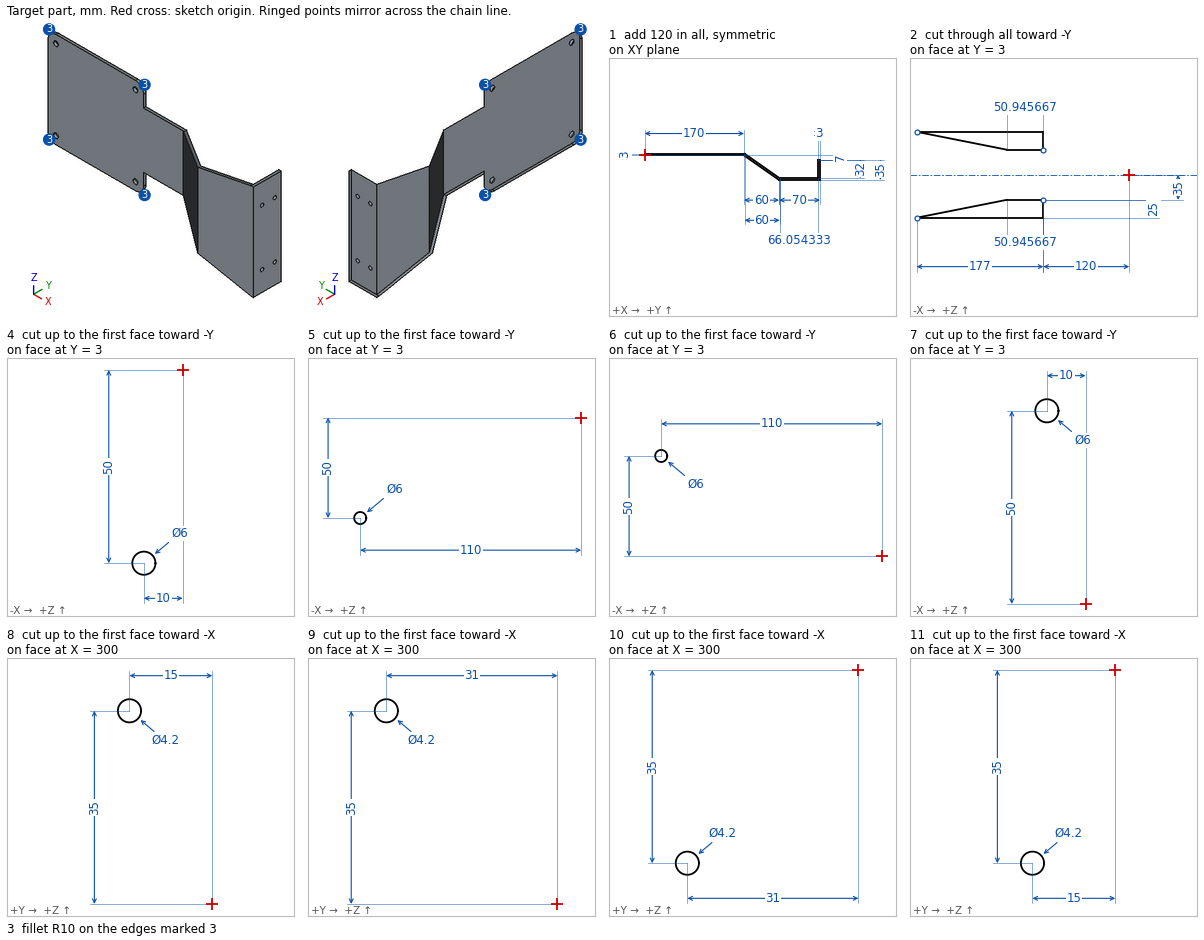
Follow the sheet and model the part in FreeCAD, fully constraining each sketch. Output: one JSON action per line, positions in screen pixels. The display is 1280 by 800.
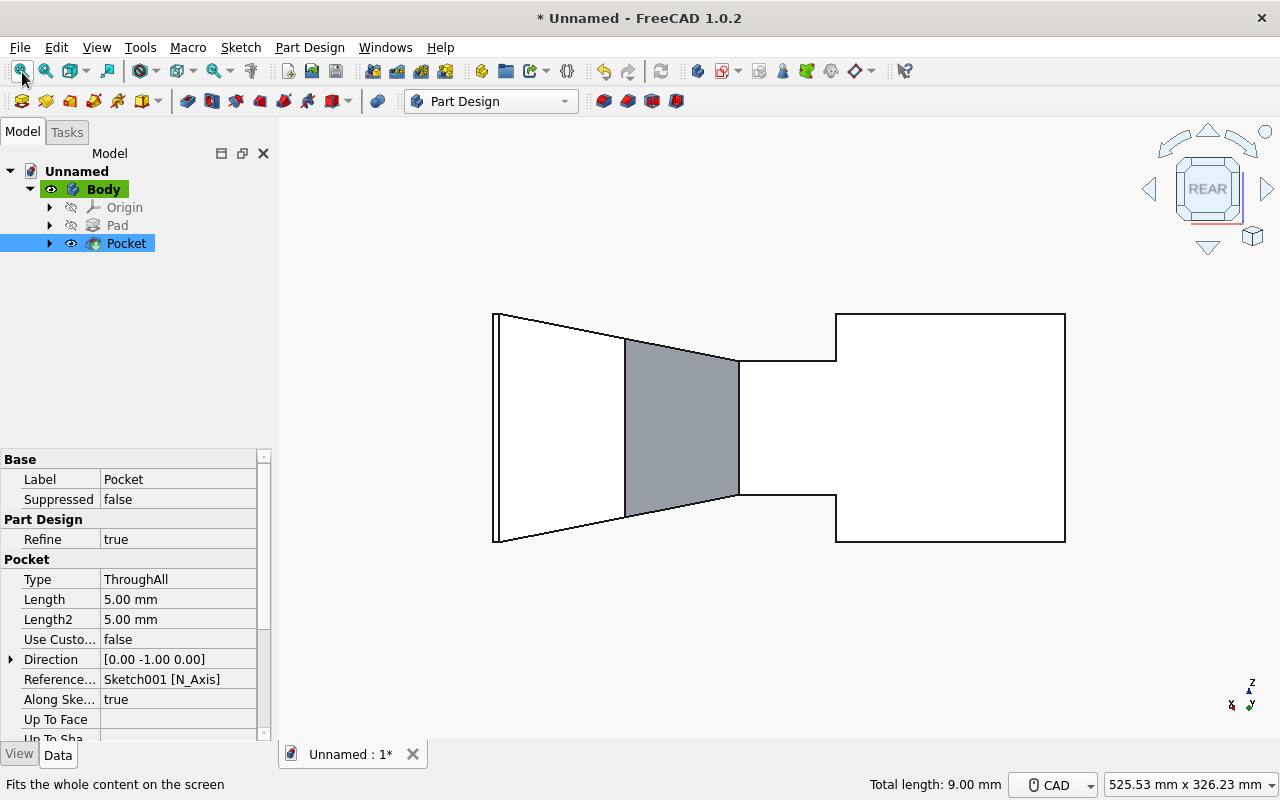
{"action": "scroll", "coordinate": [836, 313], "scroll_direction": "up", "scroll_amount": 10}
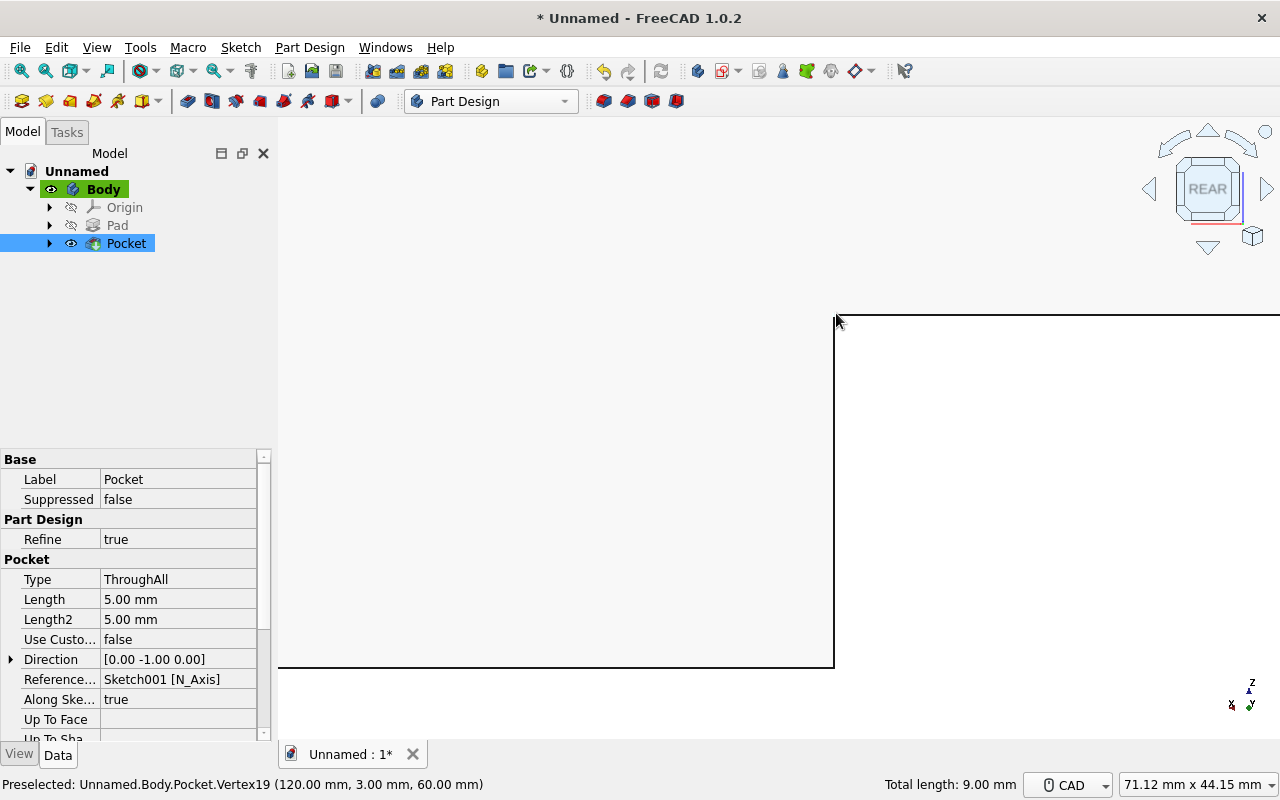
{"action": "left_click", "coordinate": [22, 72]}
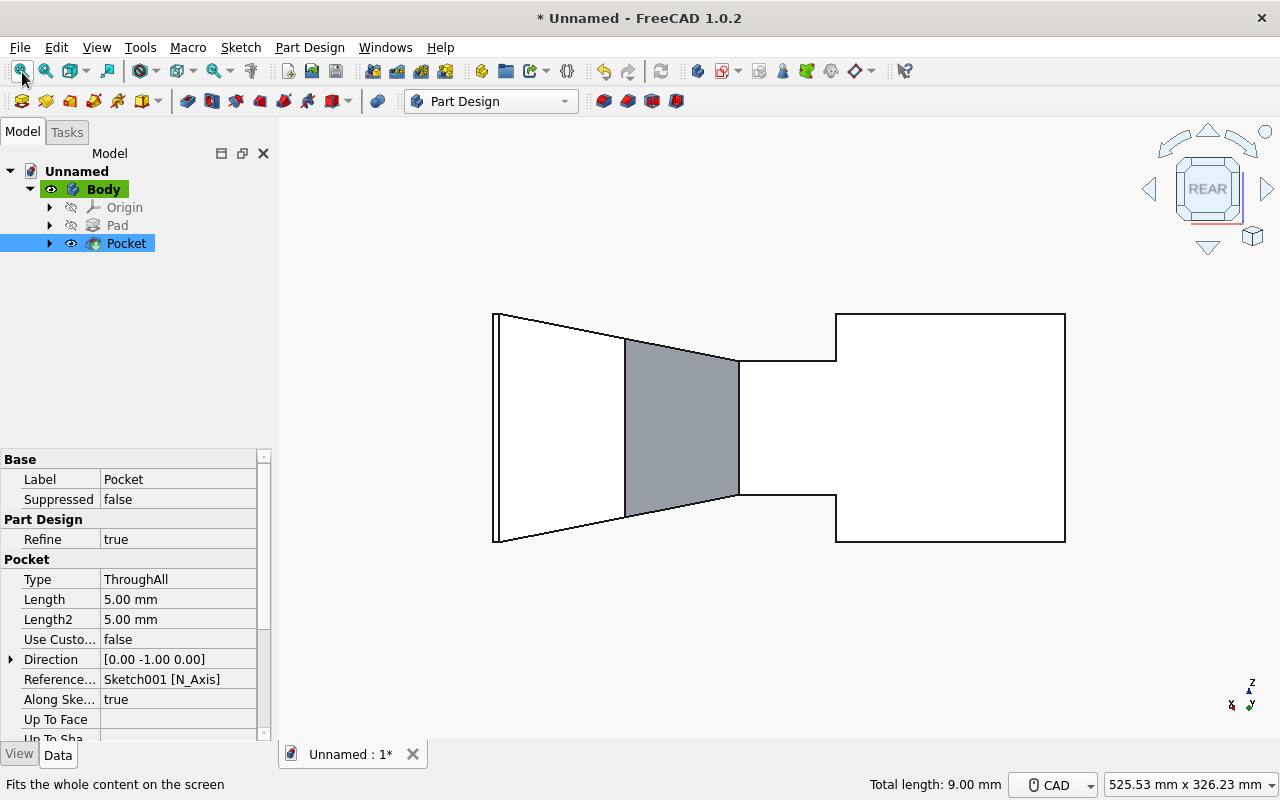
{"action": "key", "text": "6"}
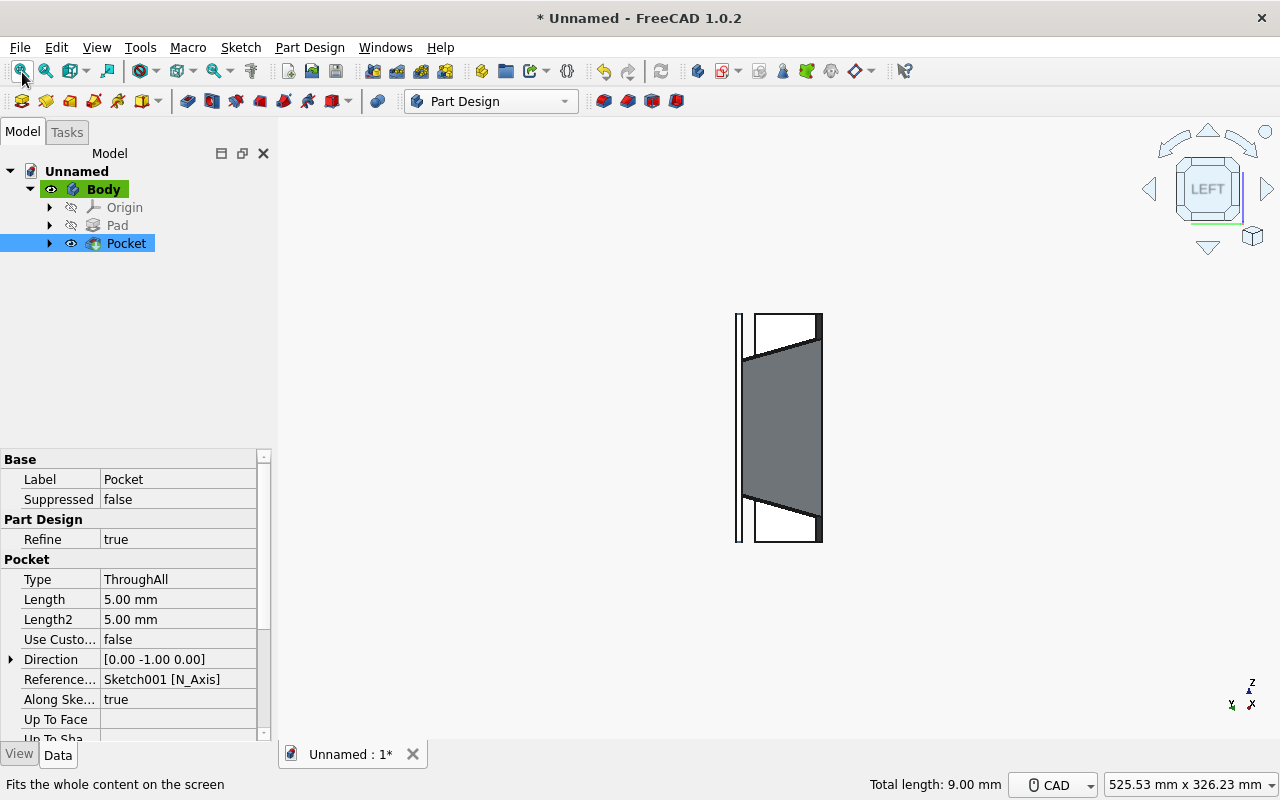
{"action": "left_click", "coordinate": [22, 72]}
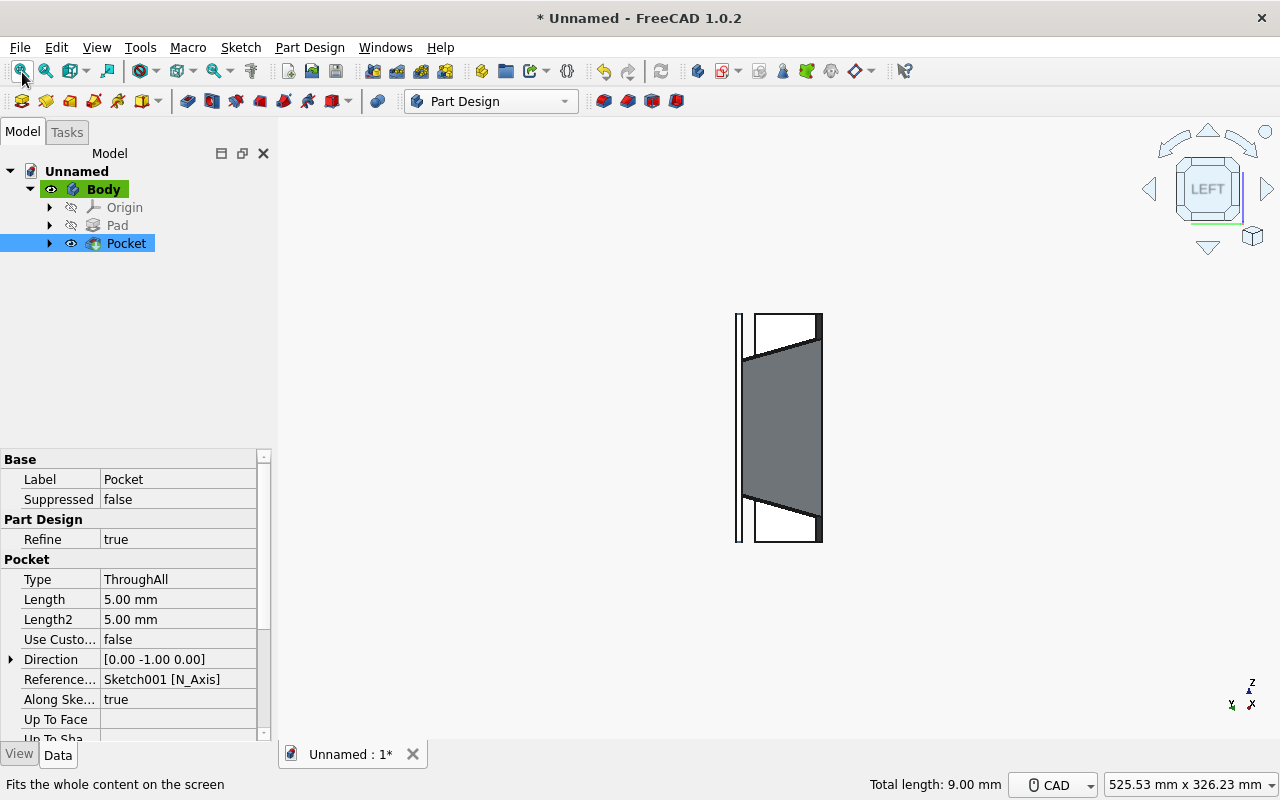
{"action": "scroll", "coordinate": [739, 313], "scroll_direction": "up", "scroll_amount": 10}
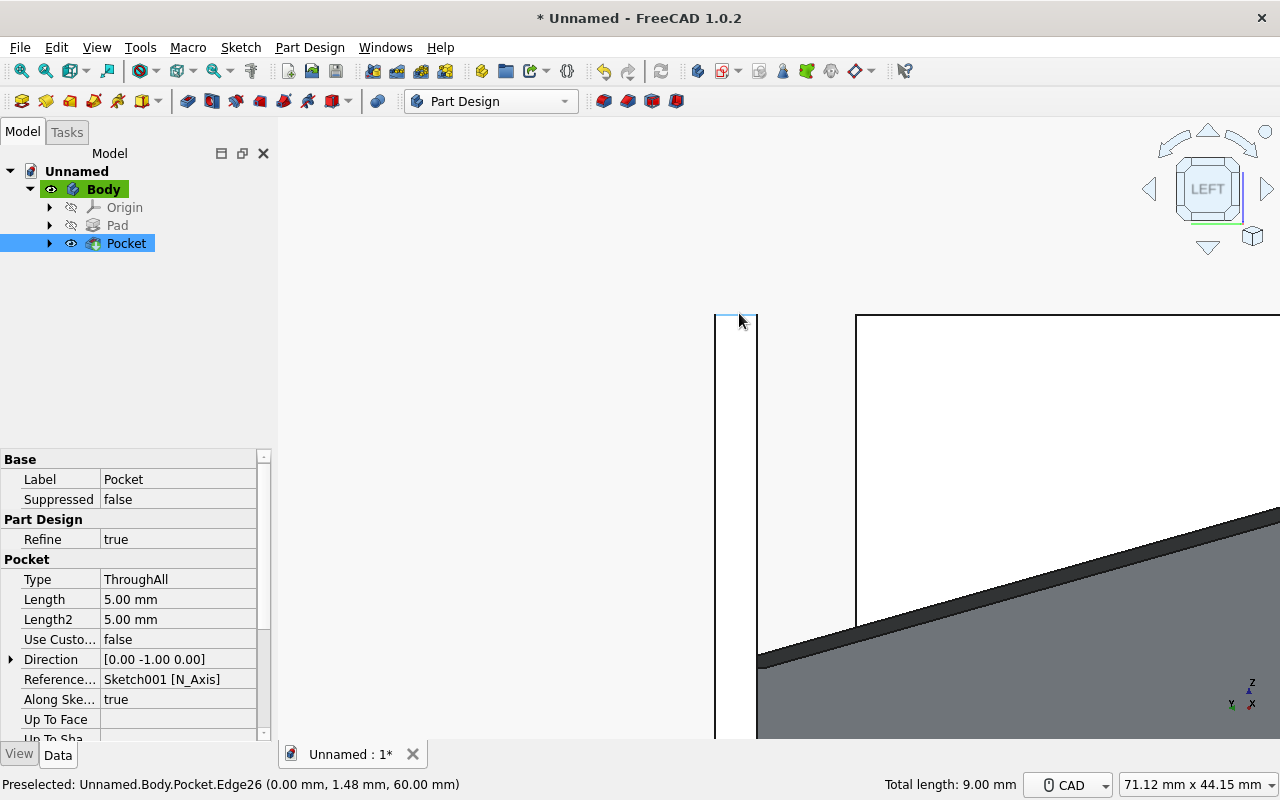
{"action": "left_click", "coordinate": [22, 72]}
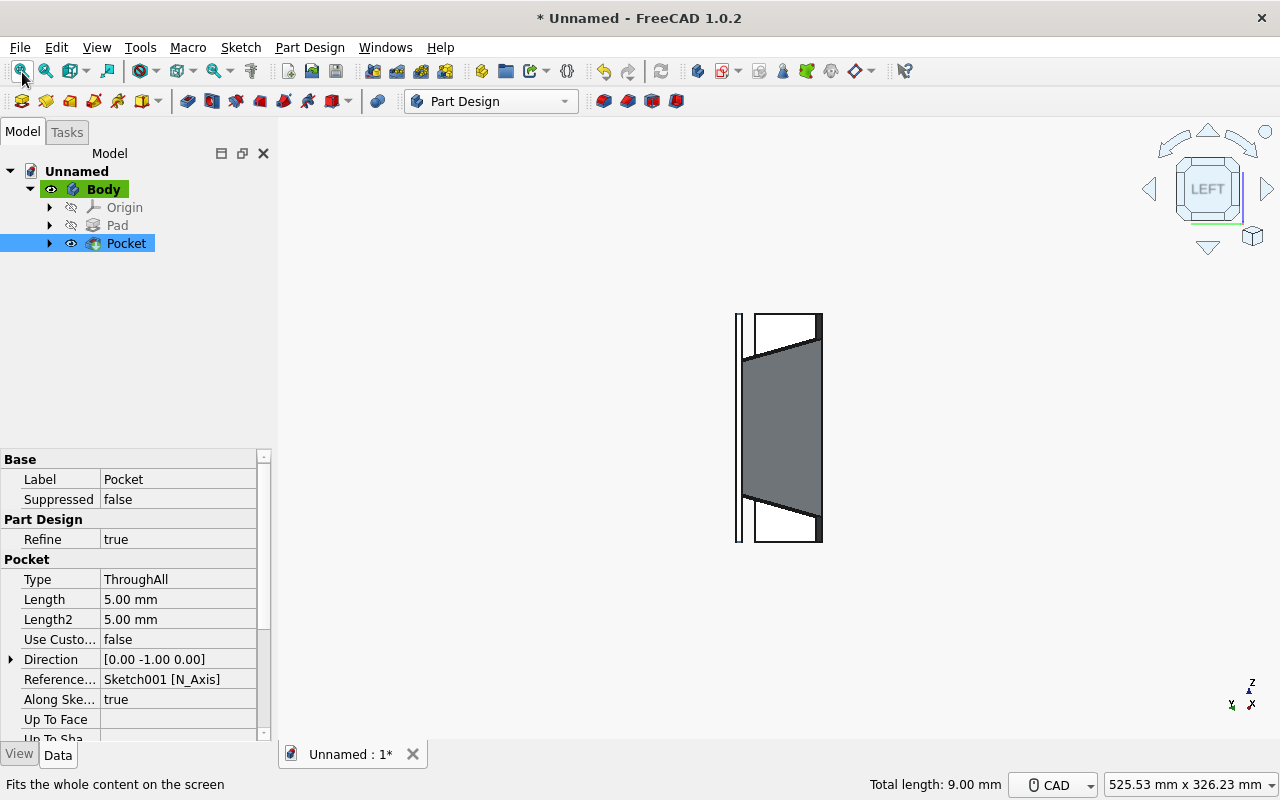
{"action": "key", "text": "v 3"}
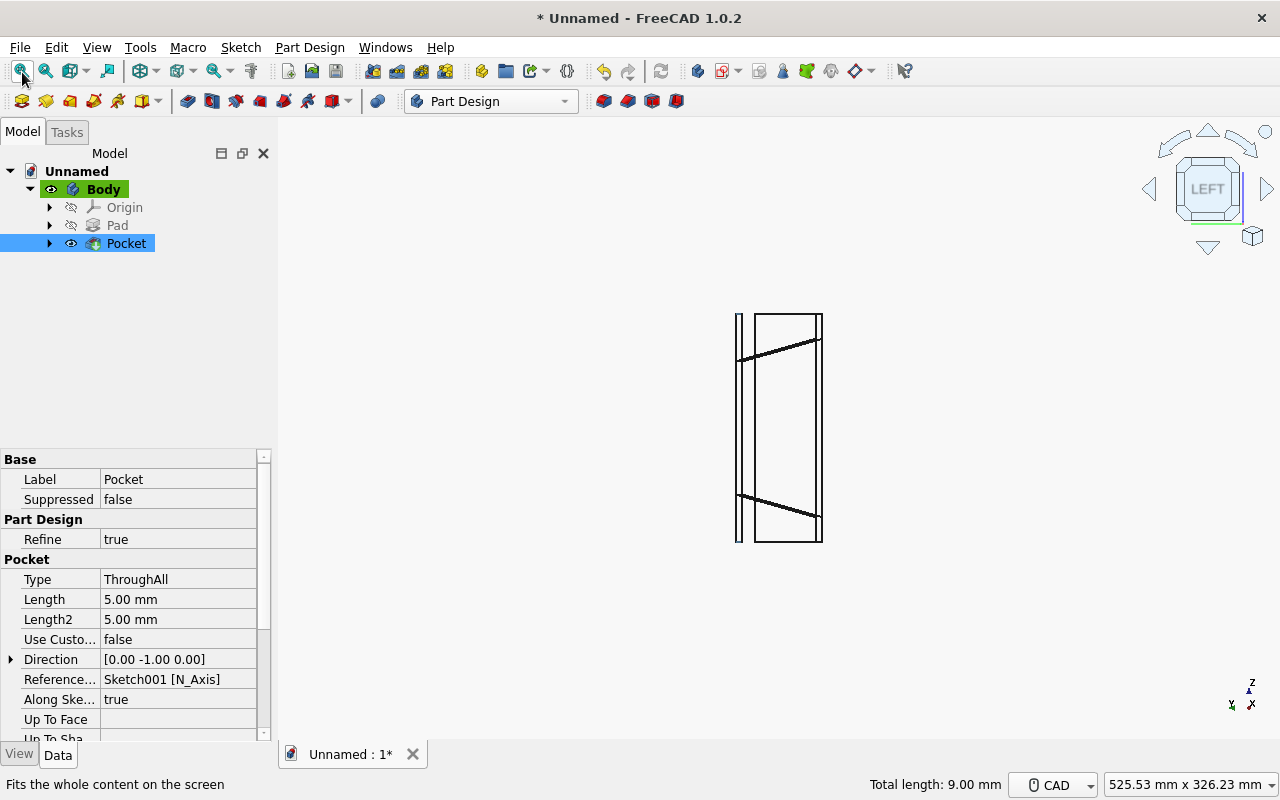
{"action": "key", "text": "0"}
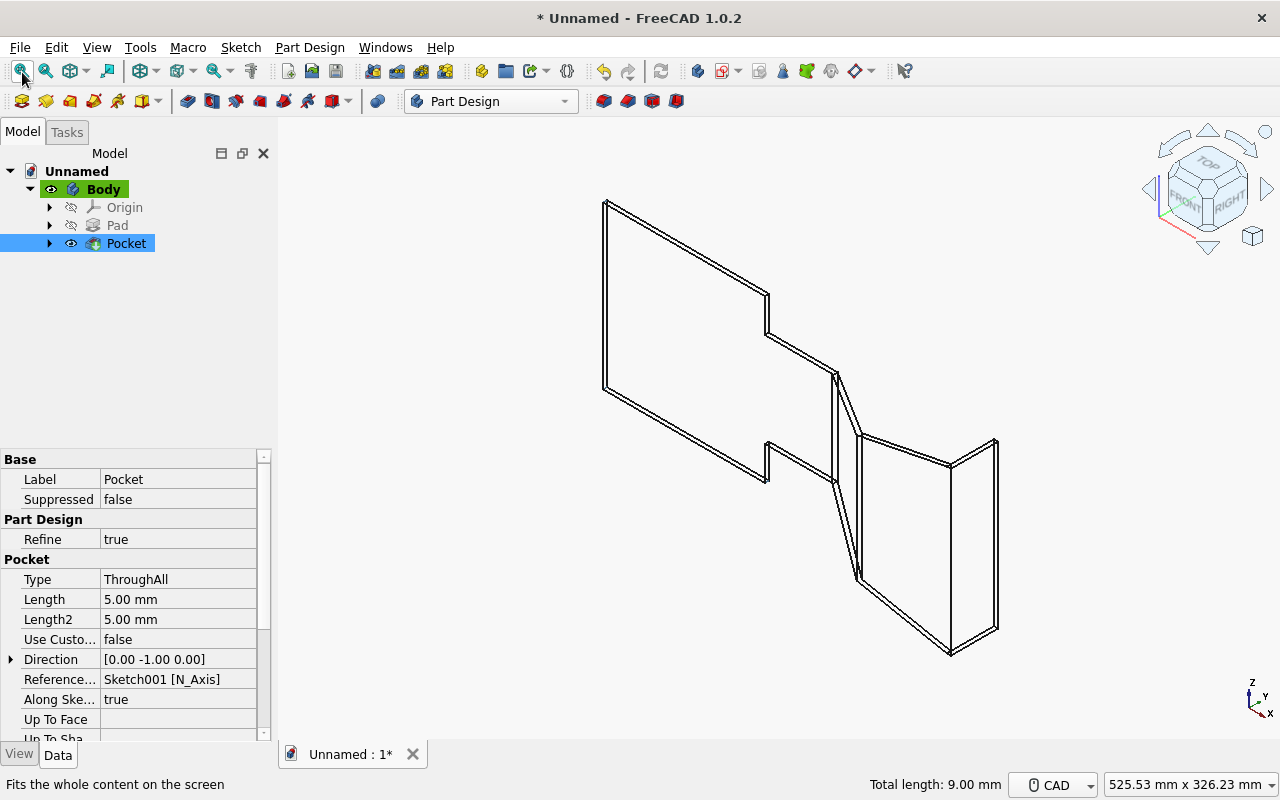
{"action": "scroll", "coordinate": [767, 294], "scroll_direction": "up", "scroll_amount": 10}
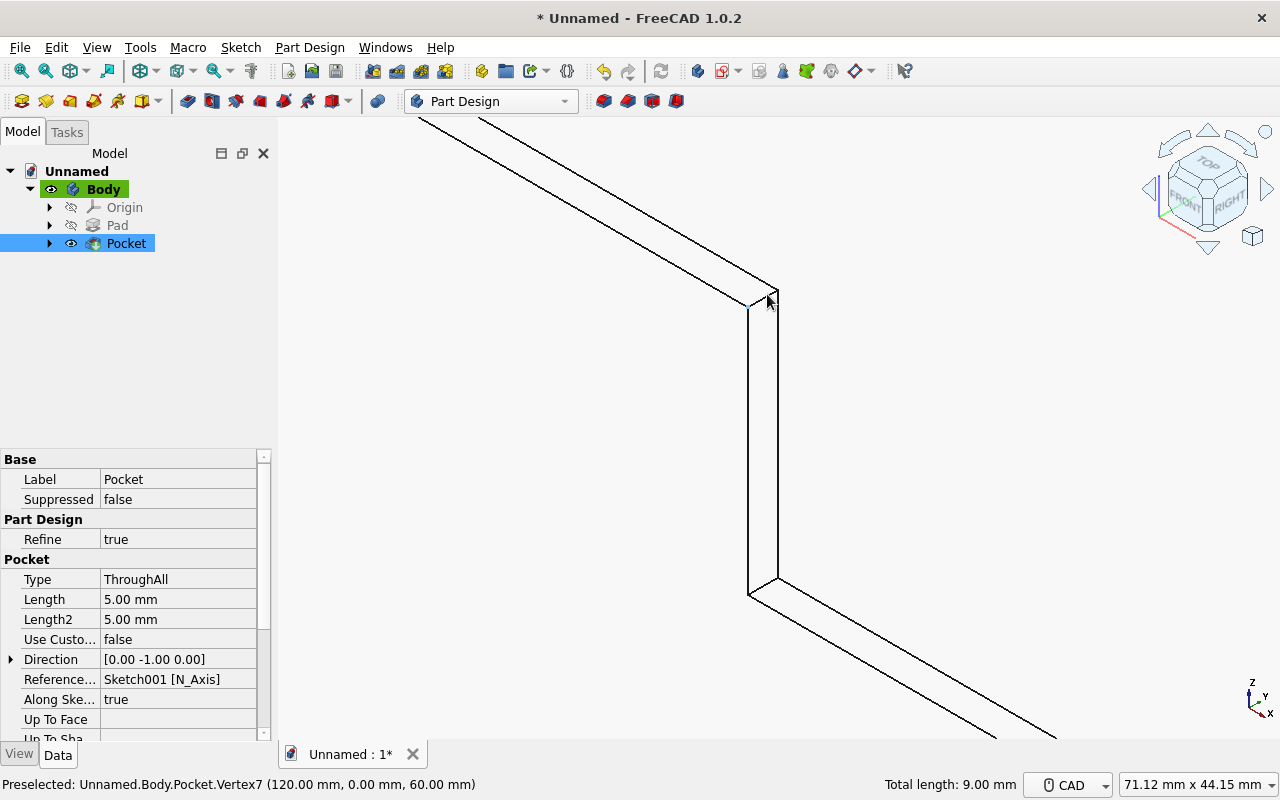
{"action": "left_click", "coordinate": [763, 298], "text": "ctrl"}